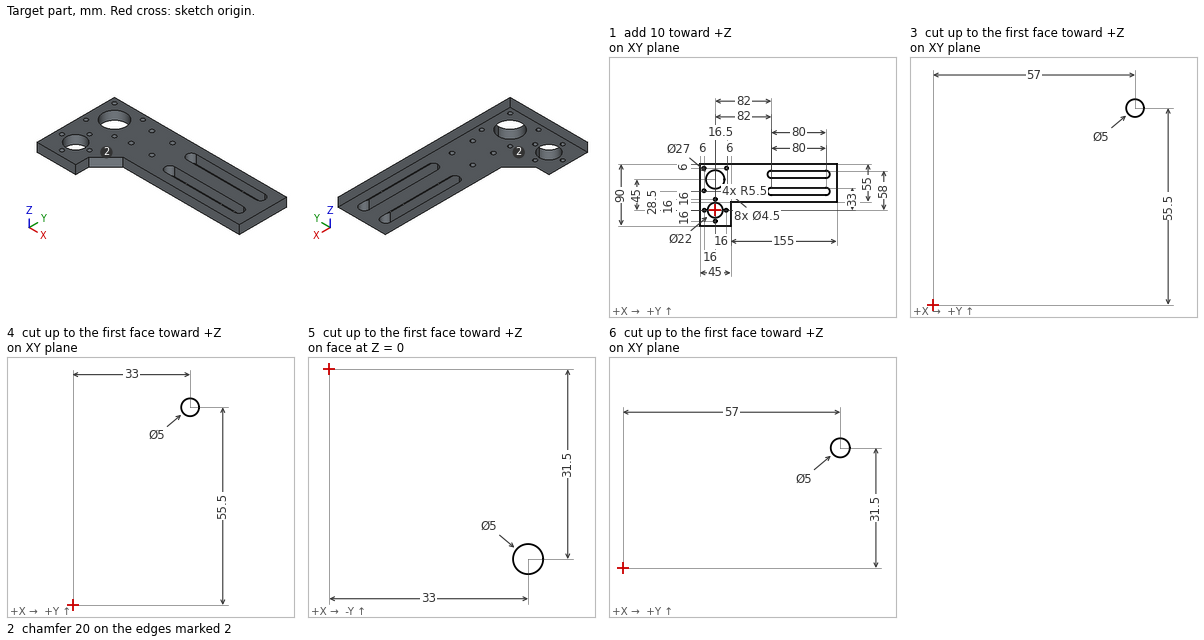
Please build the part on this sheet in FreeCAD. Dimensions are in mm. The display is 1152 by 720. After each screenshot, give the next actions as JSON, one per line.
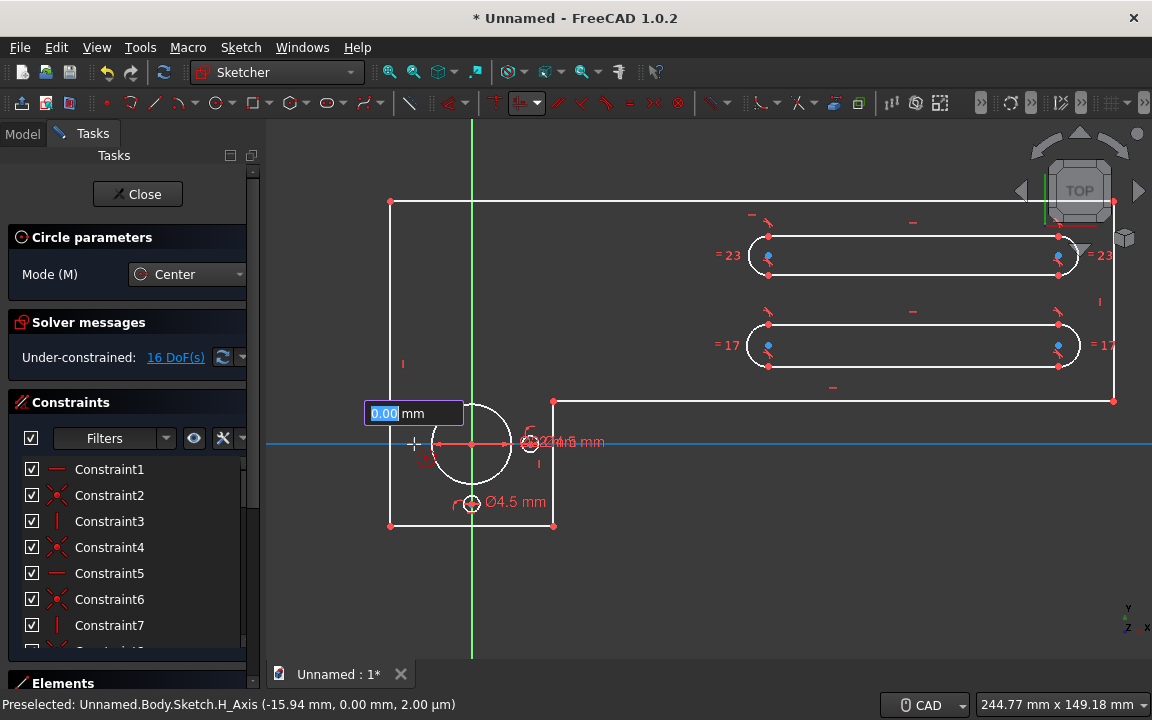
{"action": "scroll", "coordinate": [411, 452], "scroll_direction": "up", "scroll_amount": 4}
{"action": "mouse_move", "coordinate": [411, 451]}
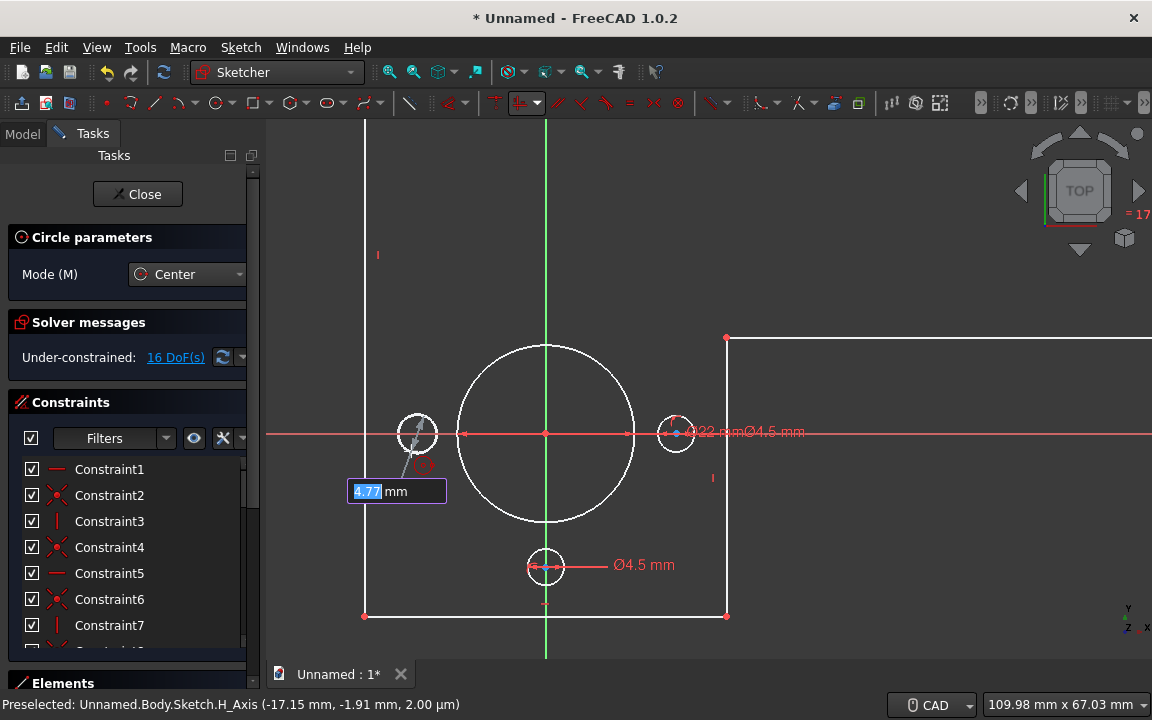
{"action": "type", "text": "4.5"}
{"action": "key", "text": "Return"}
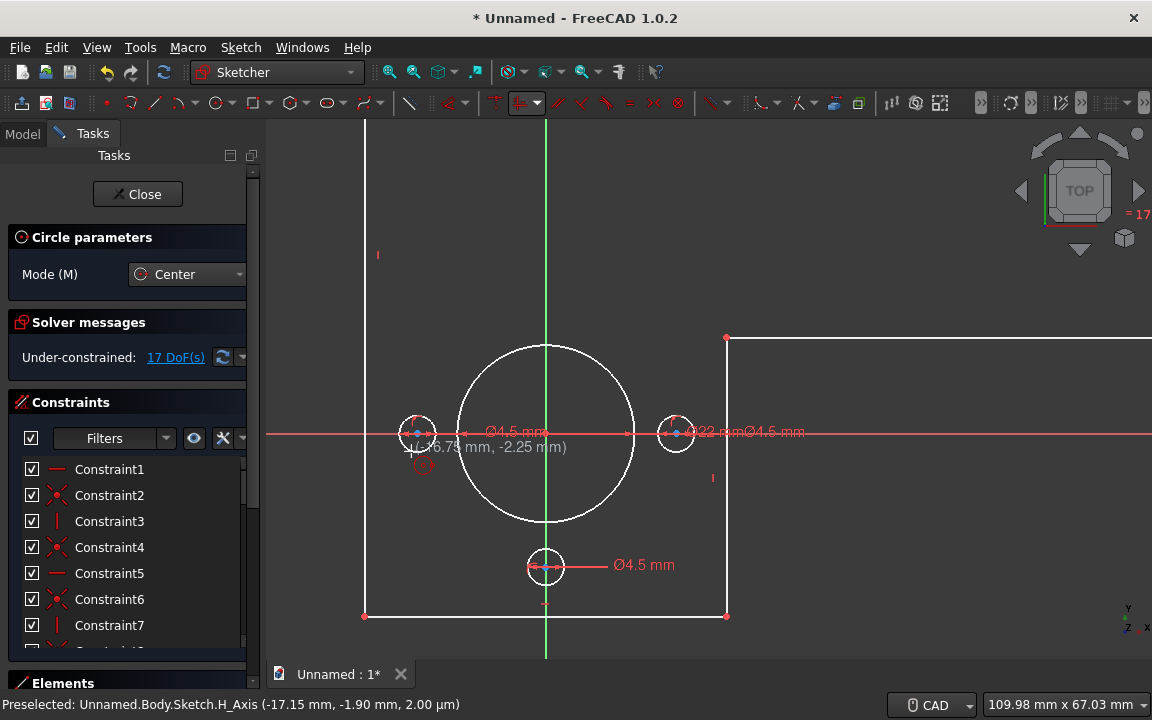
{"action": "scroll", "coordinate": [546, 305], "scroll_direction": "up", "scroll_amount": 2}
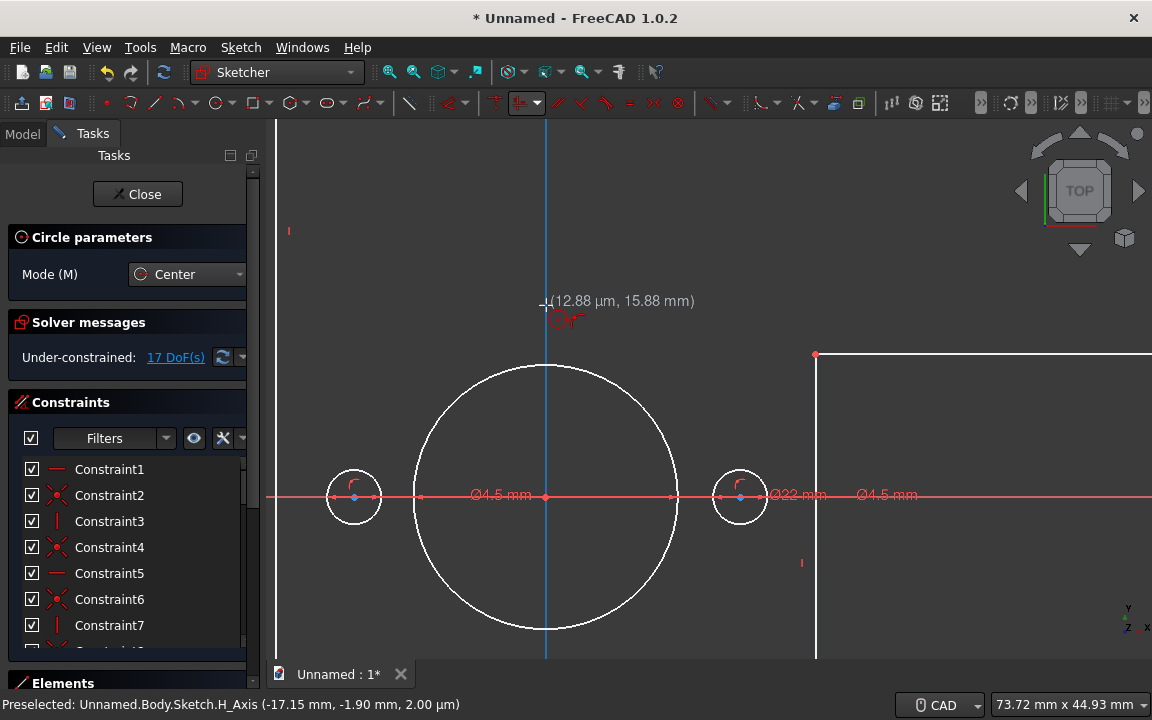
{"action": "scroll", "coordinate": [429, 430], "scroll_direction": "down", "scroll_amount": 8}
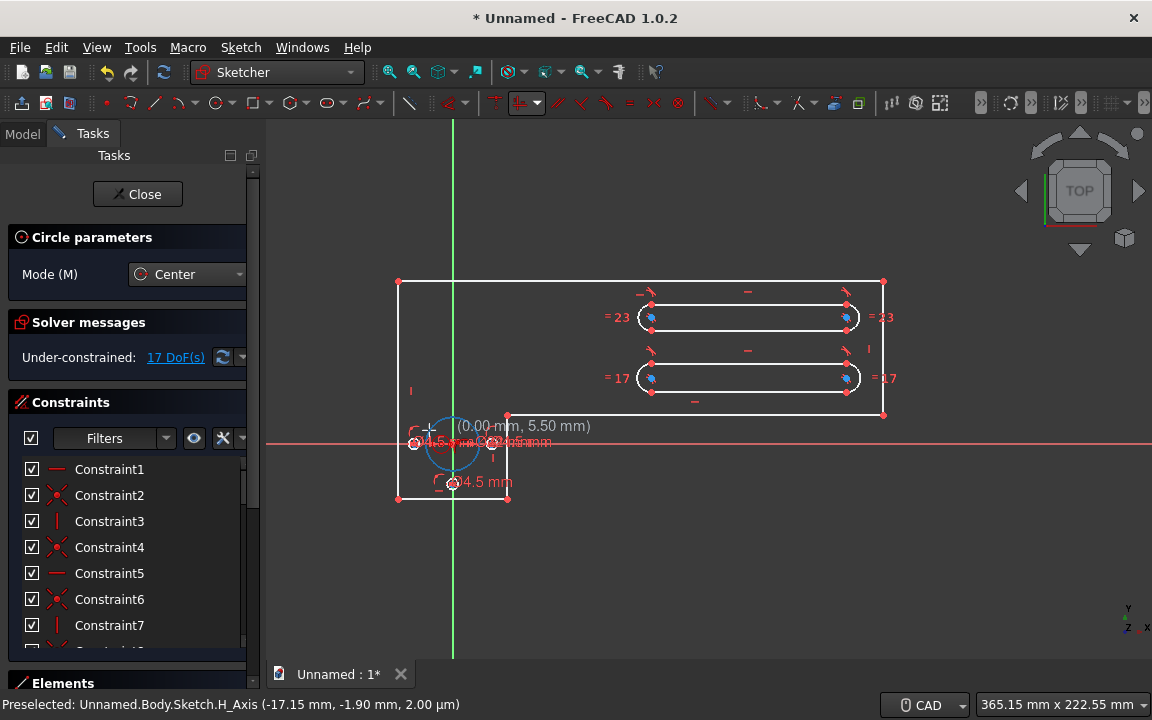
{"action": "scroll", "coordinate": [453, 405], "scroll_direction": "up", "scroll_amount": 2}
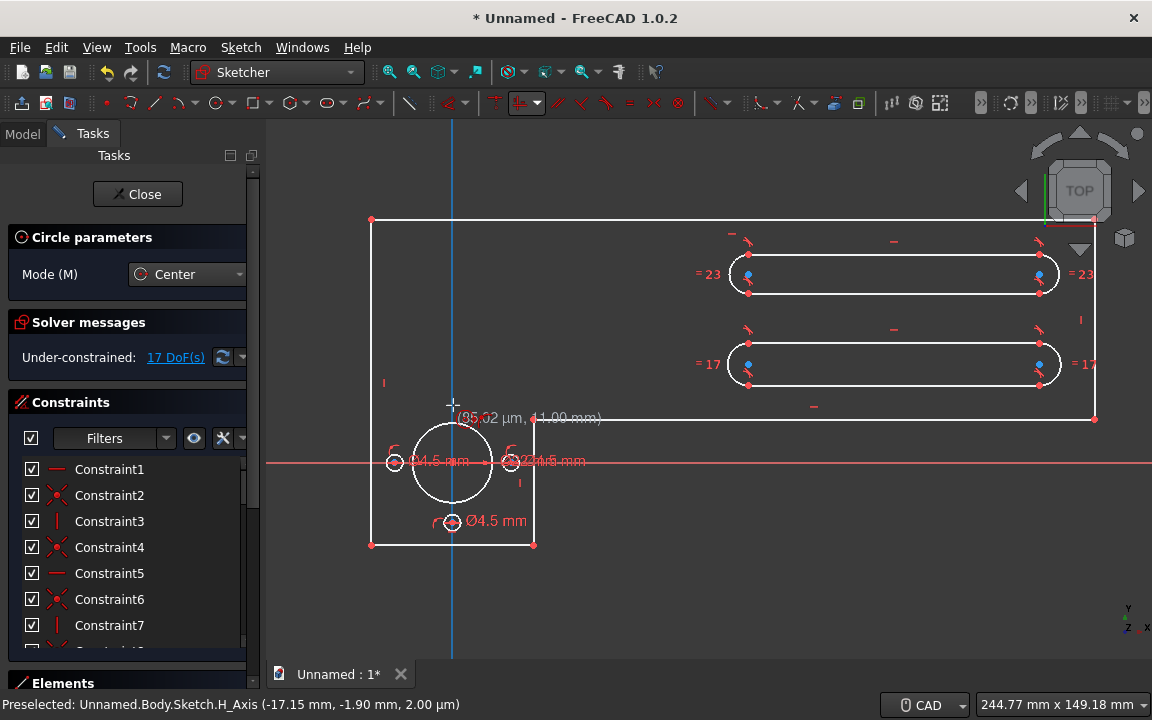
{"action": "left_click", "coordinate": [452, 405]}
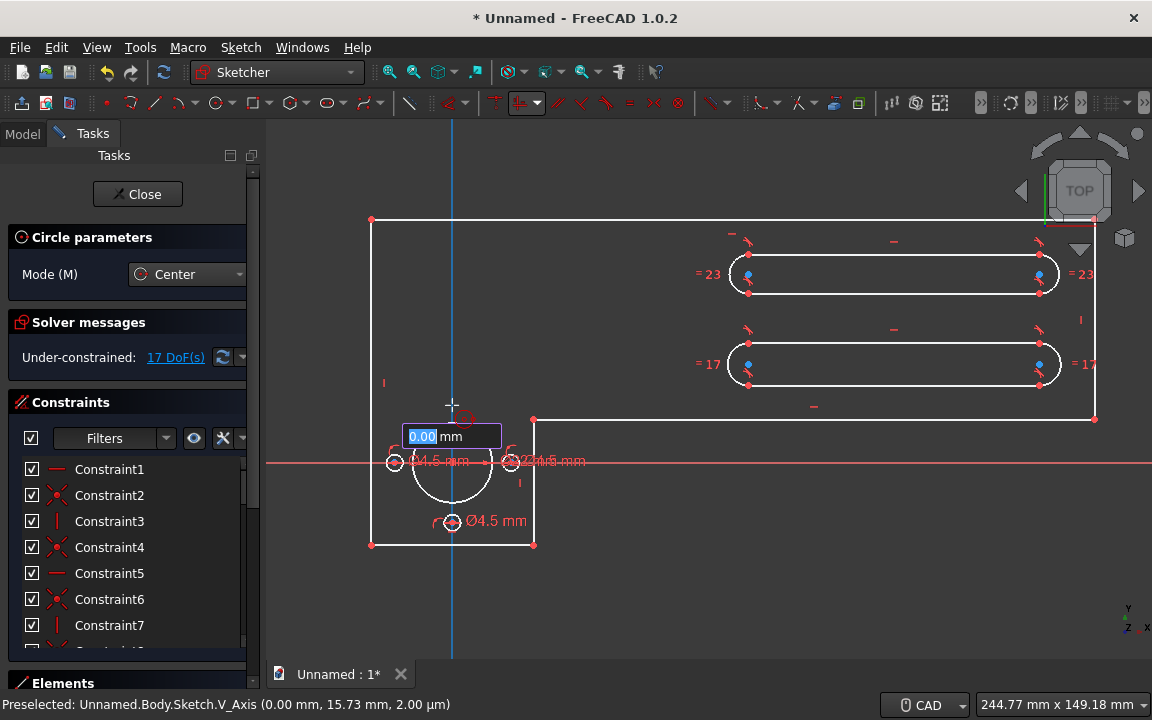
{"action": "scroll", "coordinate": [460, 402], "scroll_direction": "up", "scroll_amount": 4}
{"action": "mouse_move", "coordinate": [460, 402]}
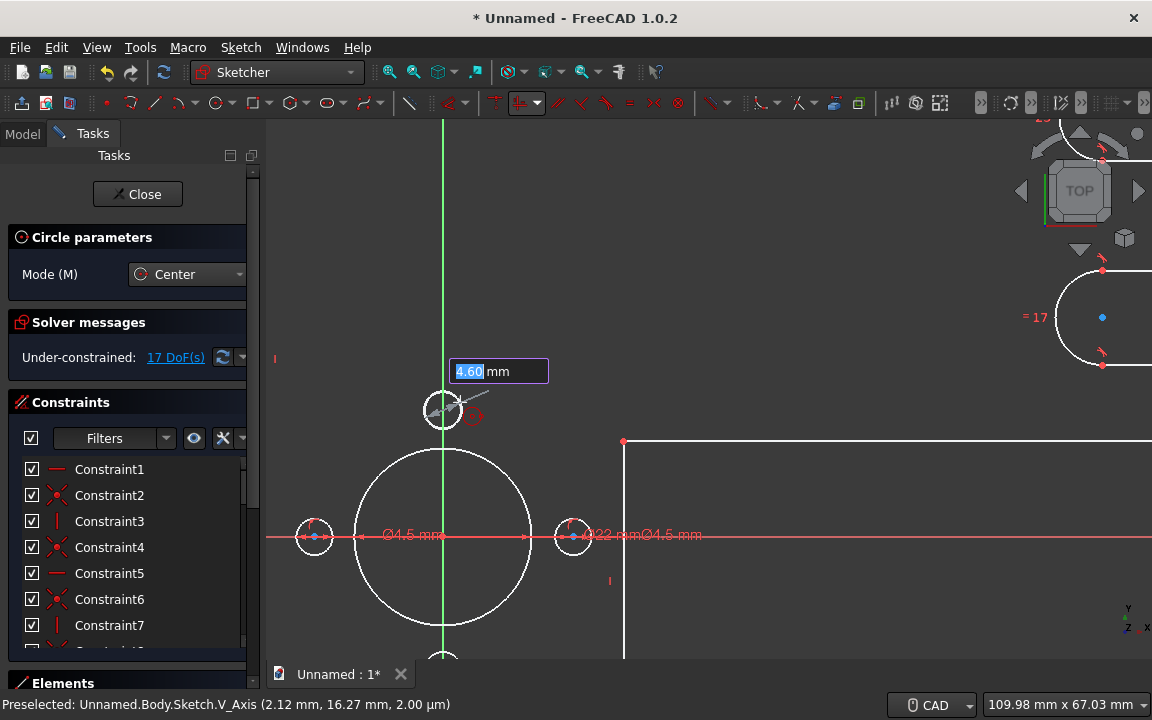
{"action": "type", "text": "4.5"}
{"action": "key", "text": "Return"}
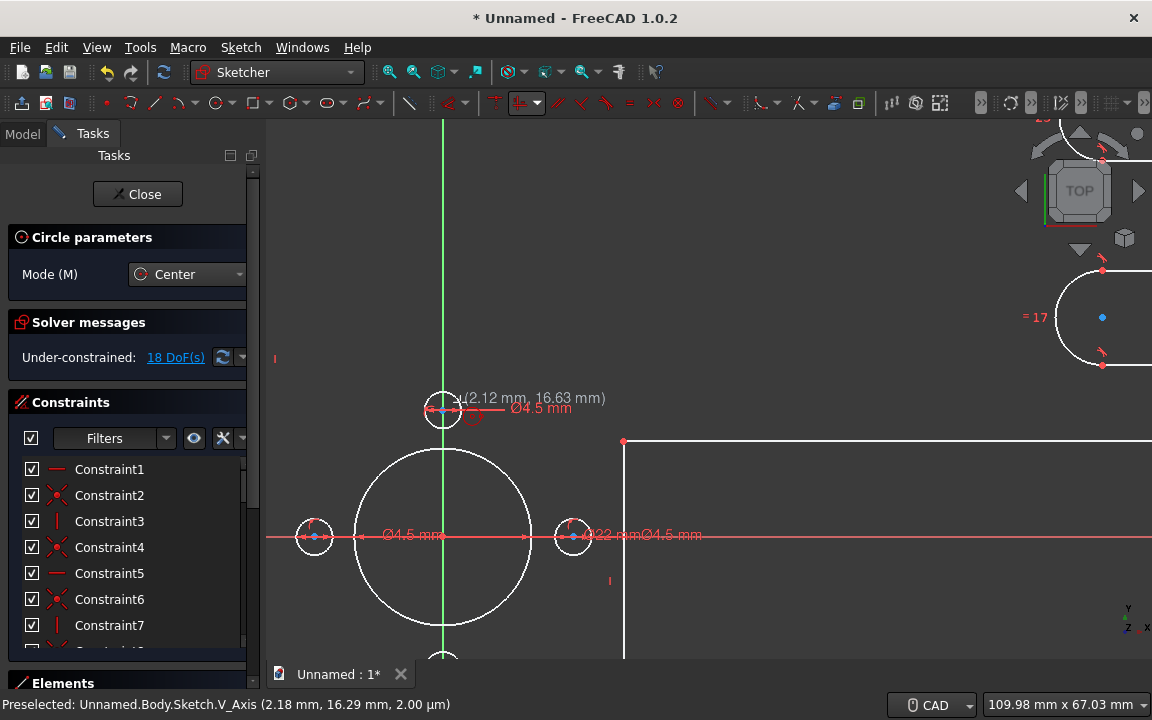
{"action": "scroll", "coordinate": [576, 307], "scroll_direction": "up", "scroll_amount": 2}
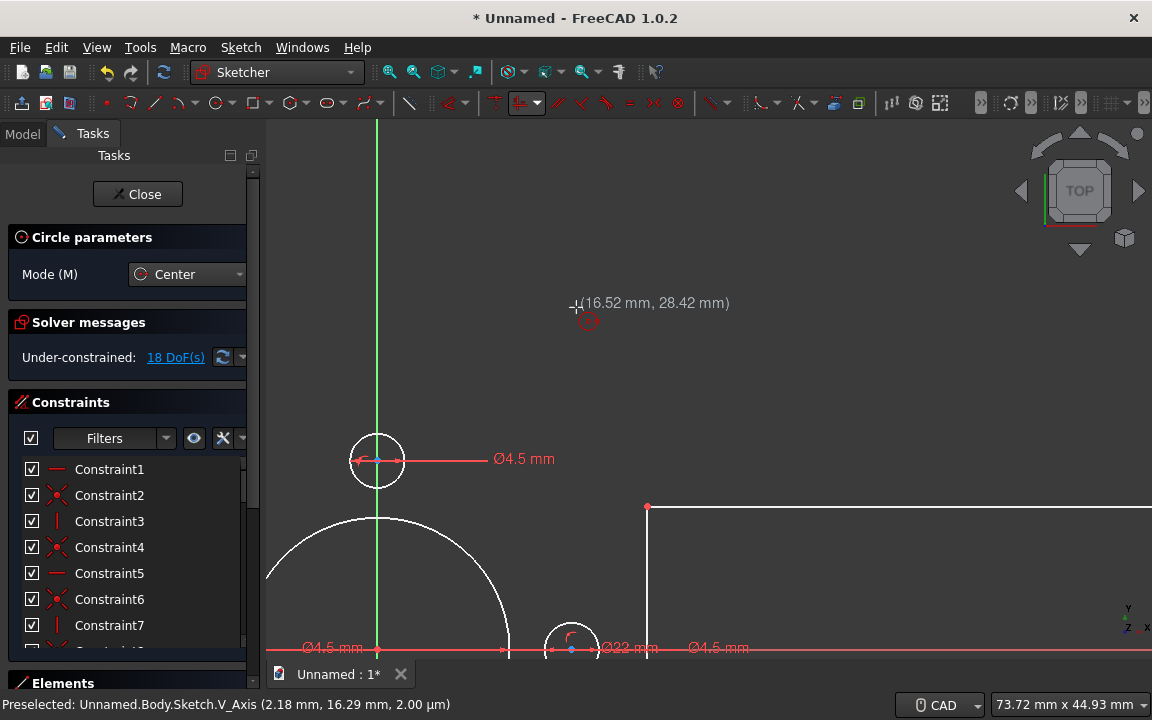
{"action": "scroll", "coordinate": [471, 391], "scroll_direction": "down", "scroll_amount": 8}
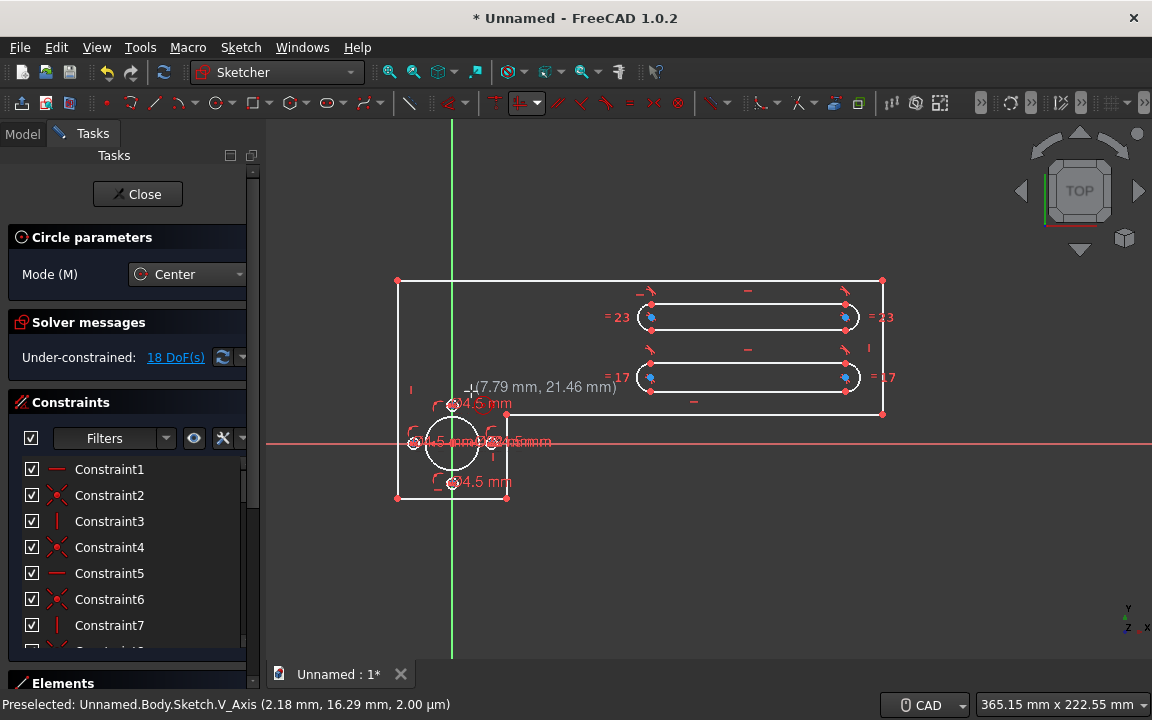
{"action": "left_click", "coordinate": [492, 375]}
{"action": "mouse_move", "coordinate": [496, 371]}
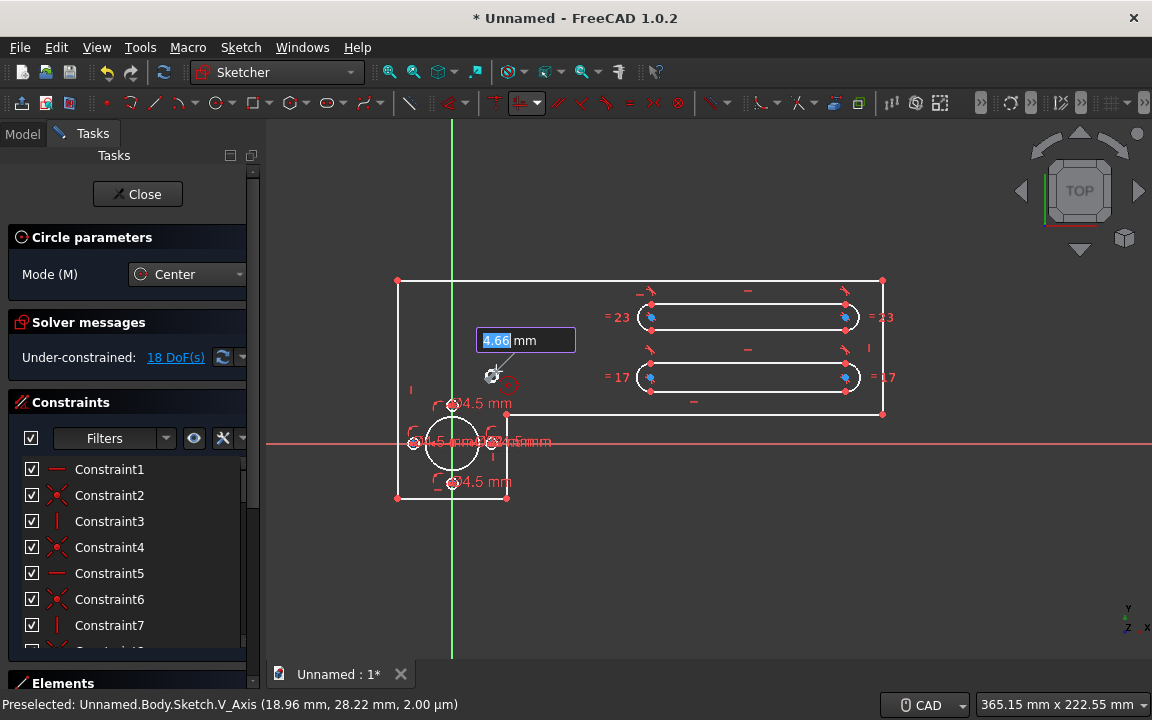
{"action": "type", "text": "4.5"}
{"action": "key", "text": "Return"}